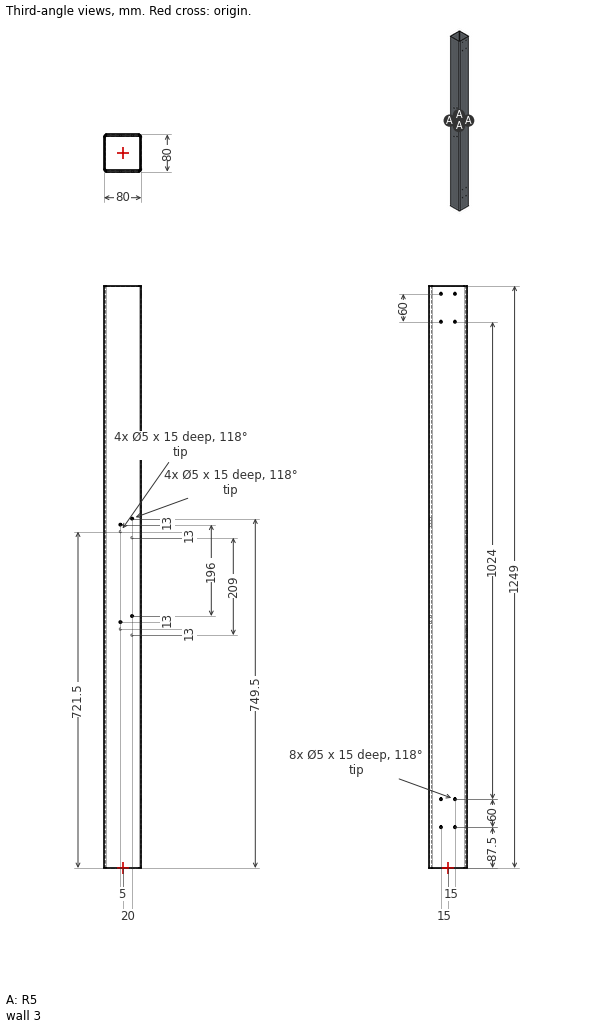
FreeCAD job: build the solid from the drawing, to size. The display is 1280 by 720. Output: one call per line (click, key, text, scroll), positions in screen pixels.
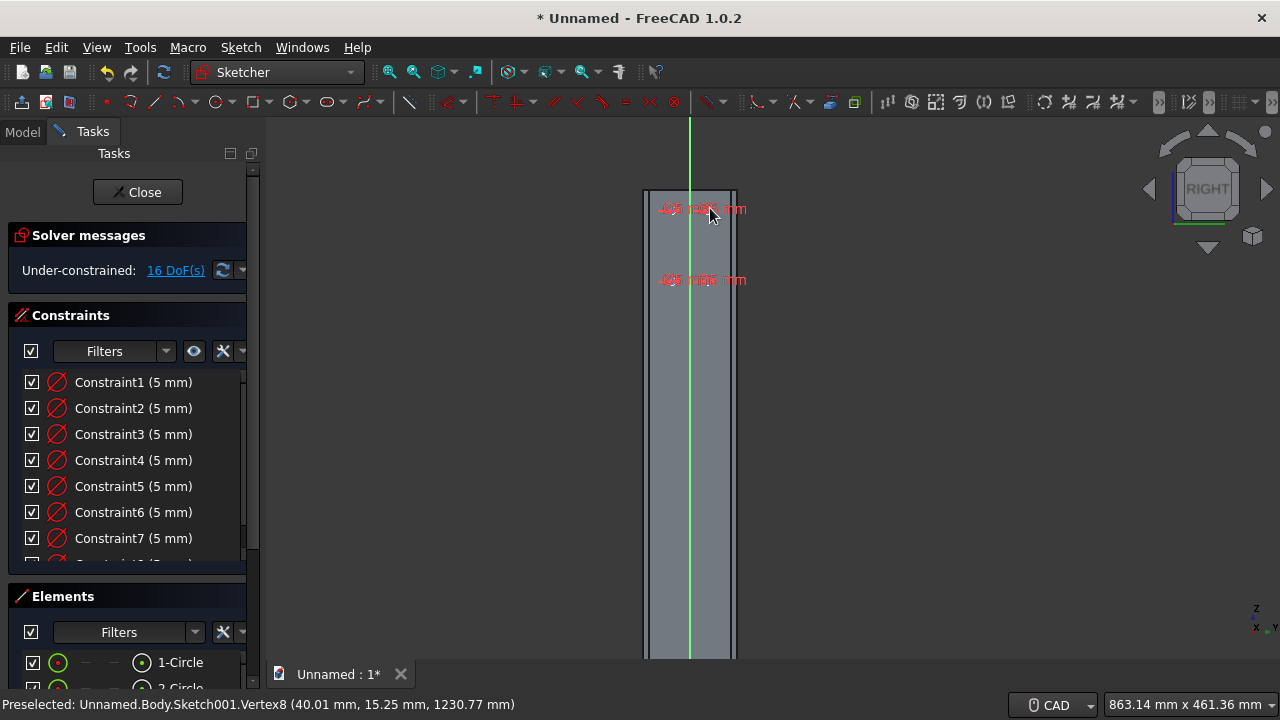
scroll(709, 210, down, 7)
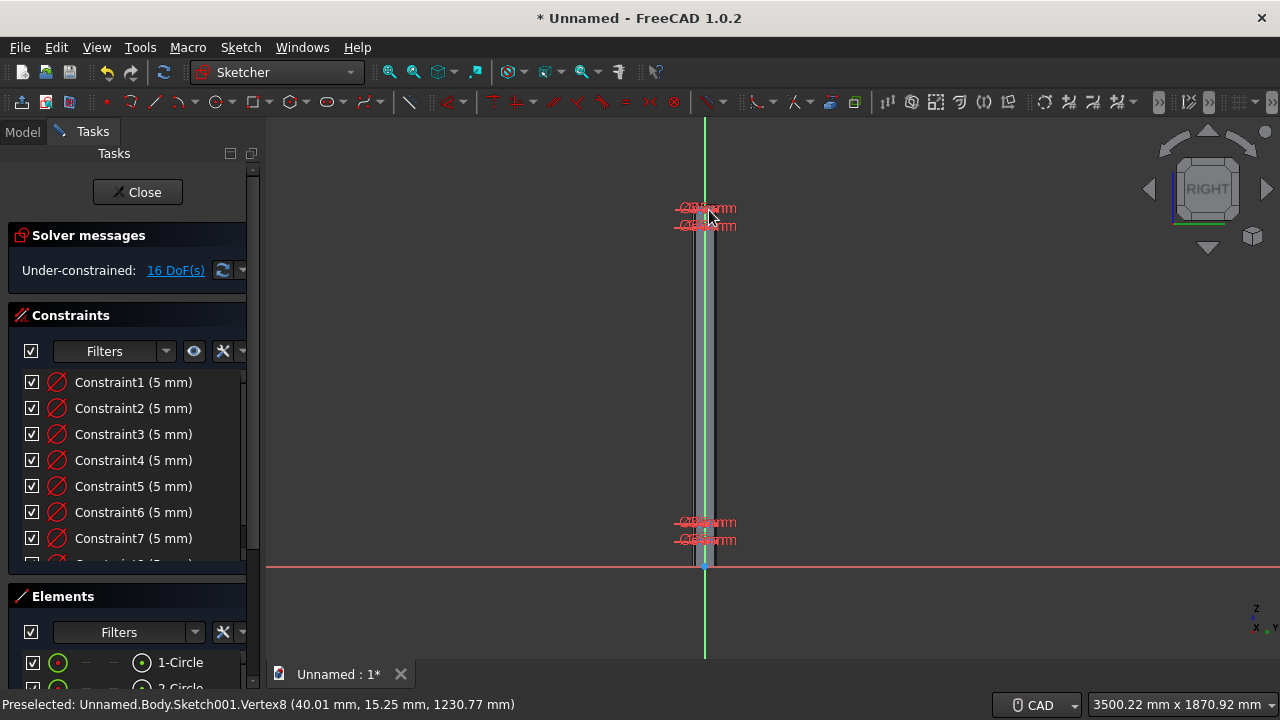
scroll(709, 525, up, 2)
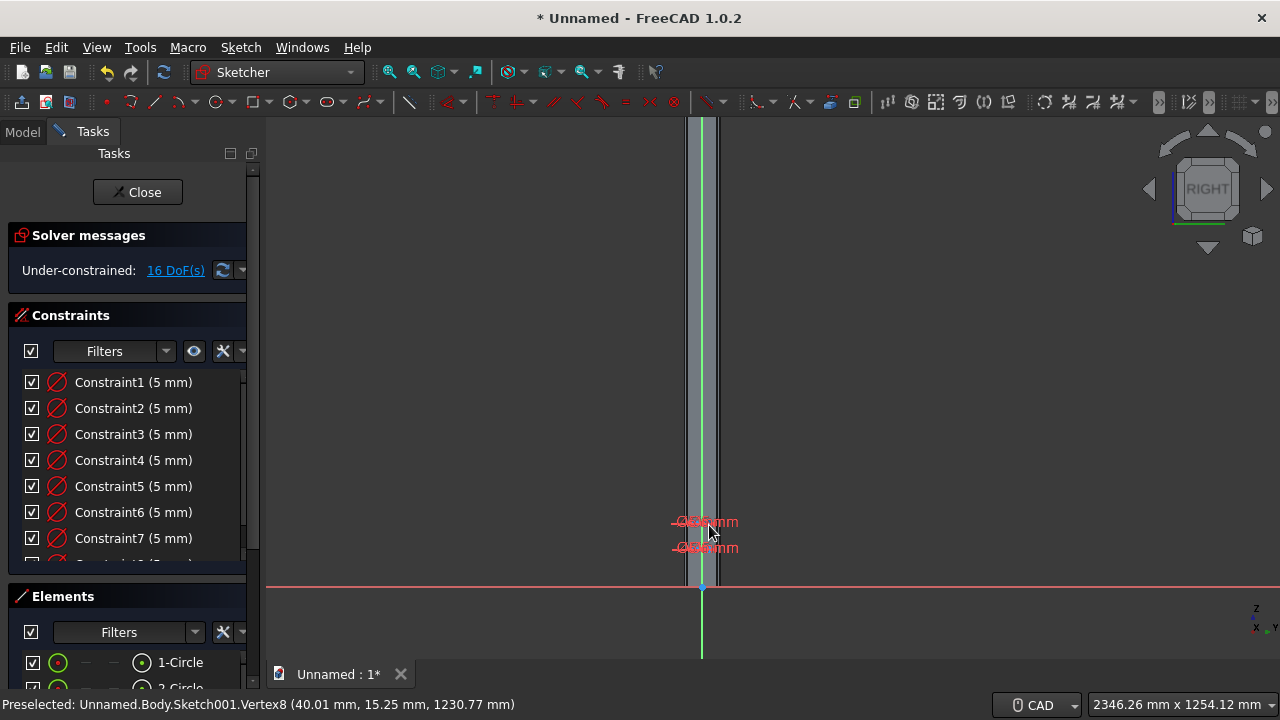
click(709, 524)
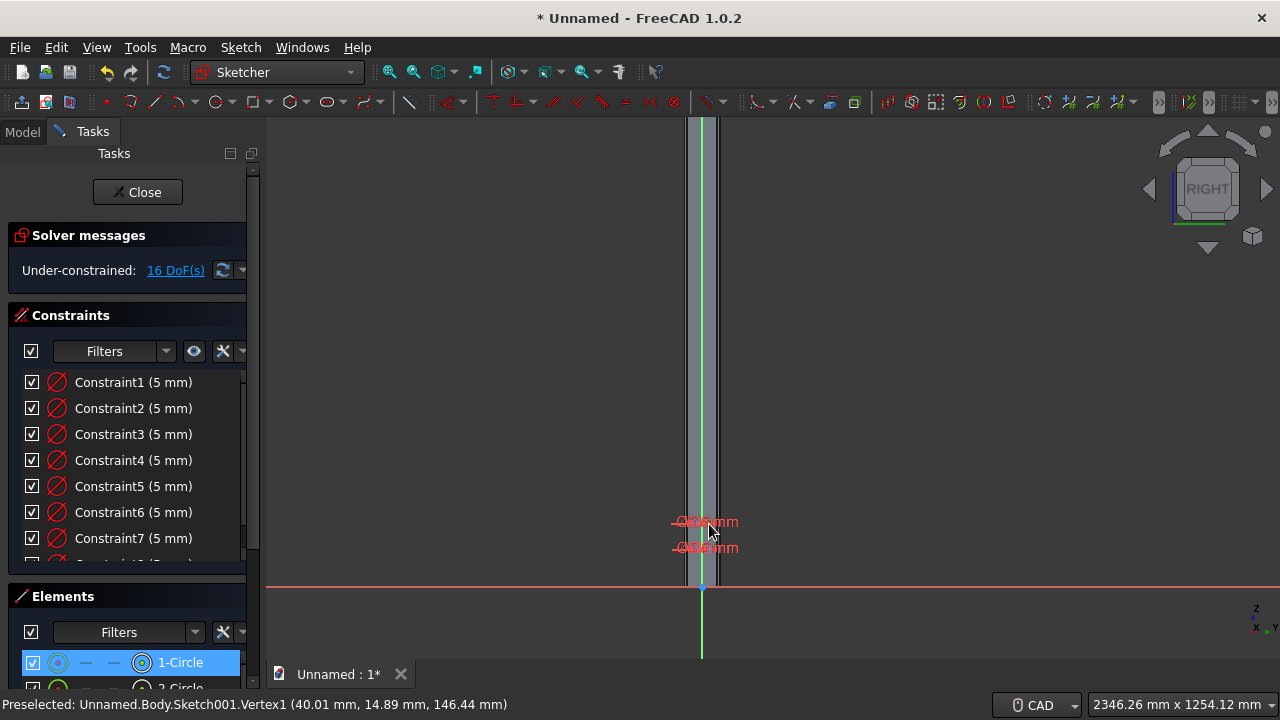
click(709, 550)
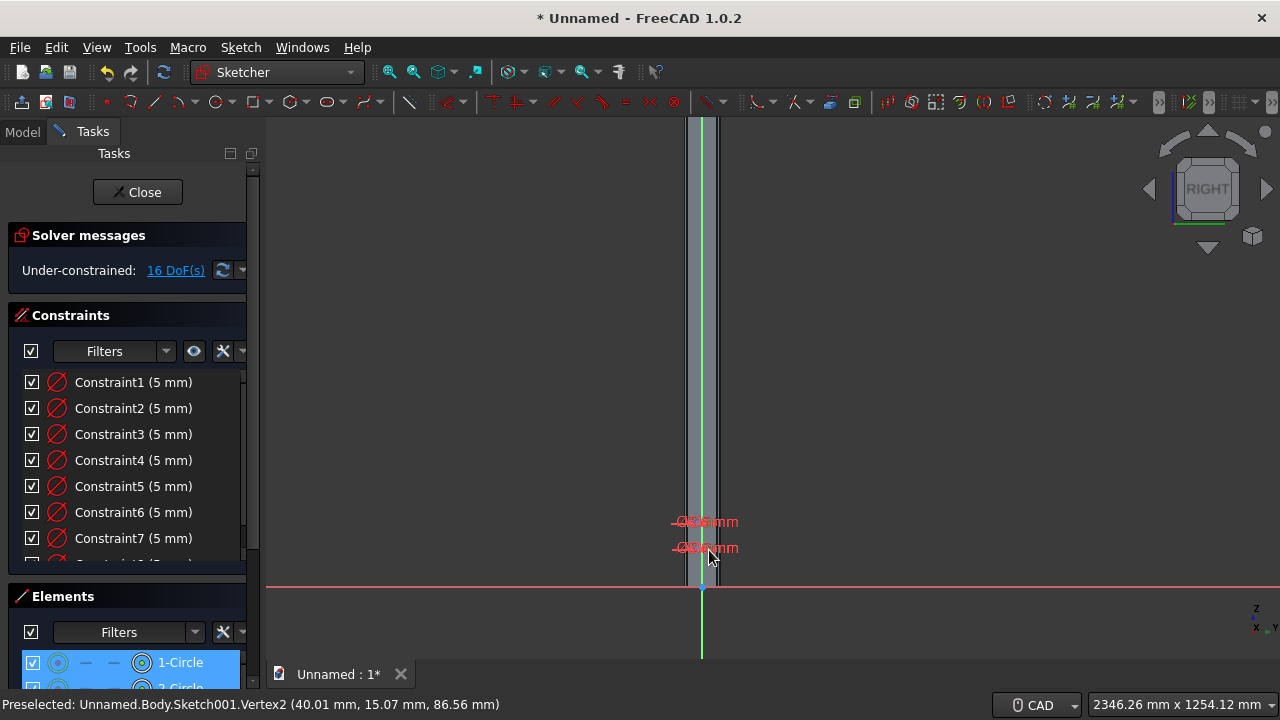
key(v)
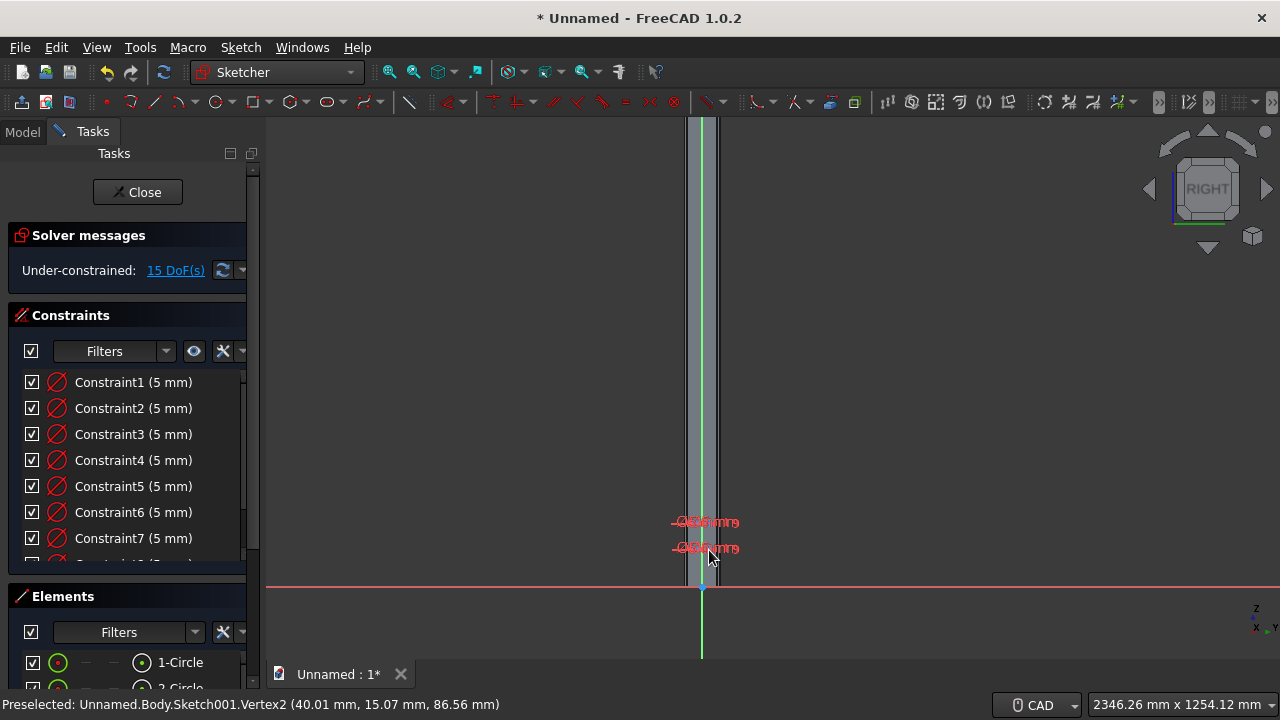
click(709, 550)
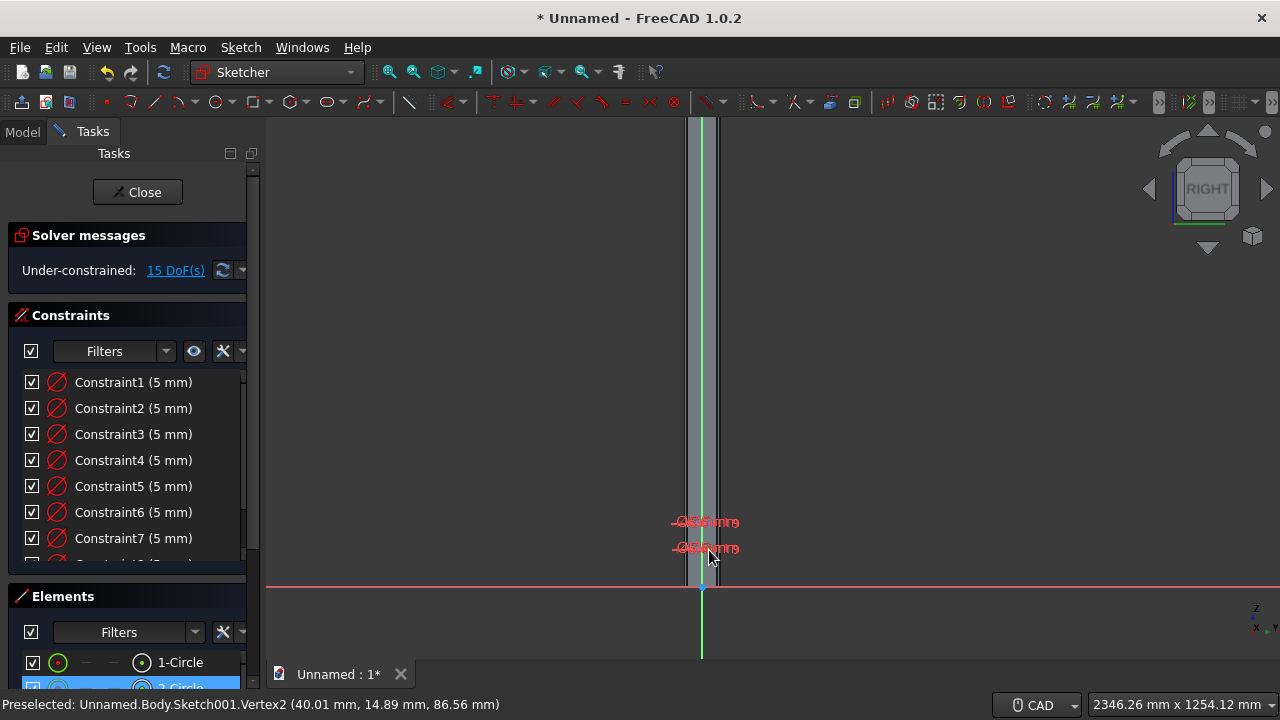
click(696, 550)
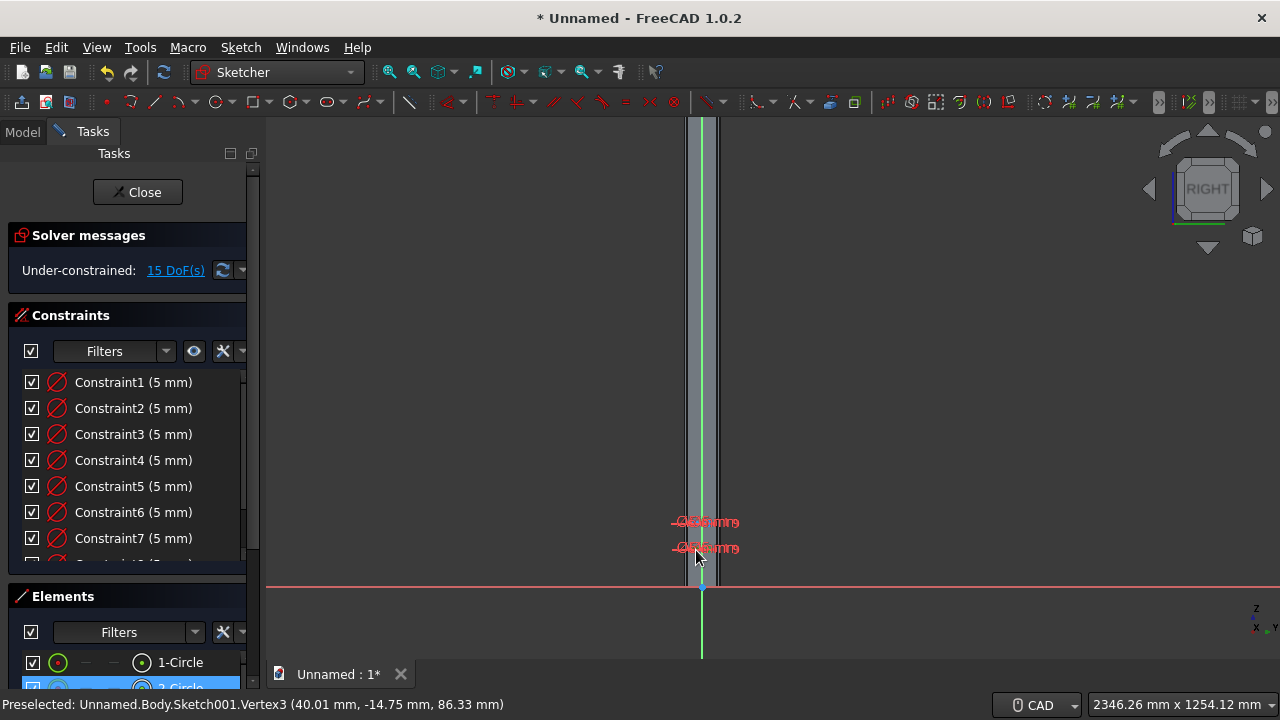
click(536, 102)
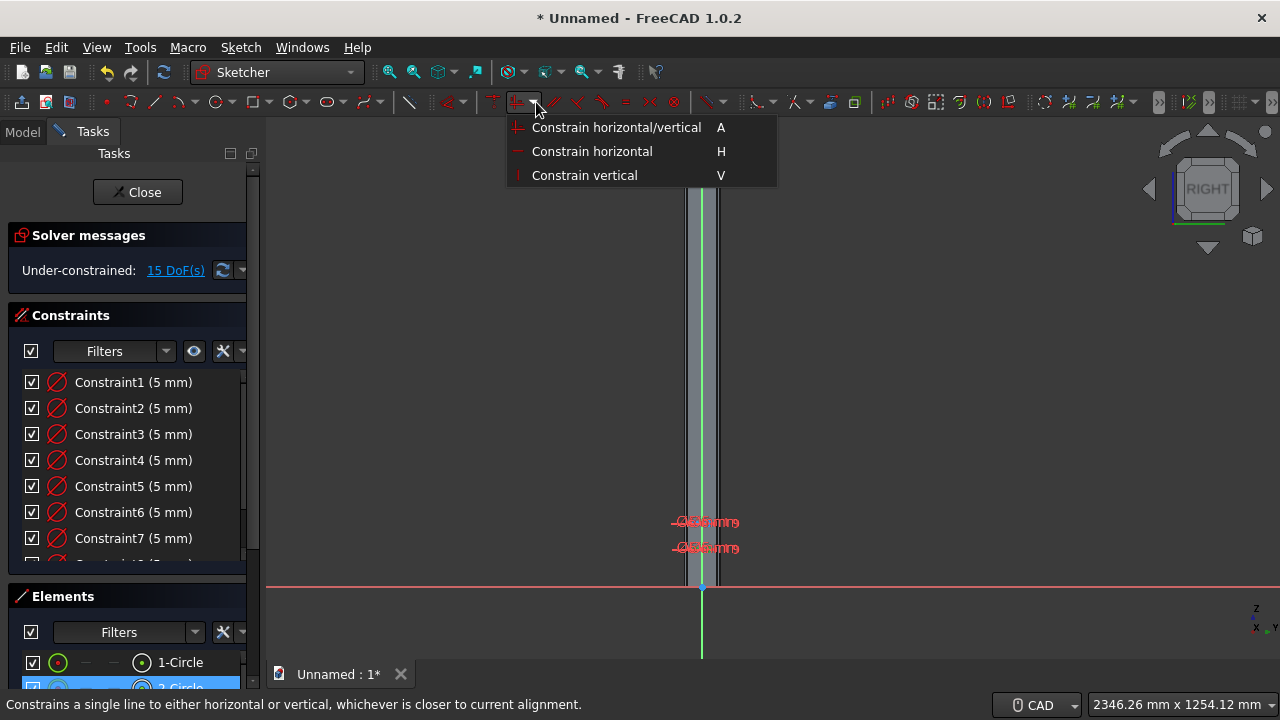
click(642, 151)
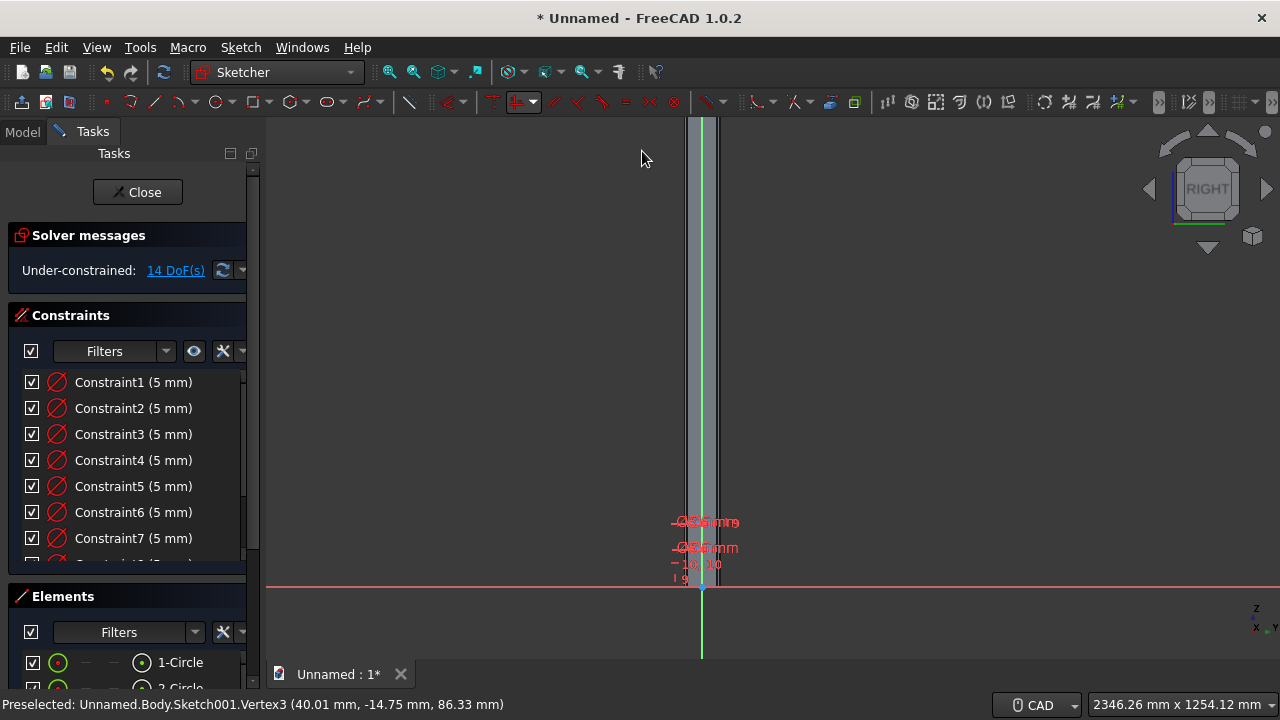
click(696, 550)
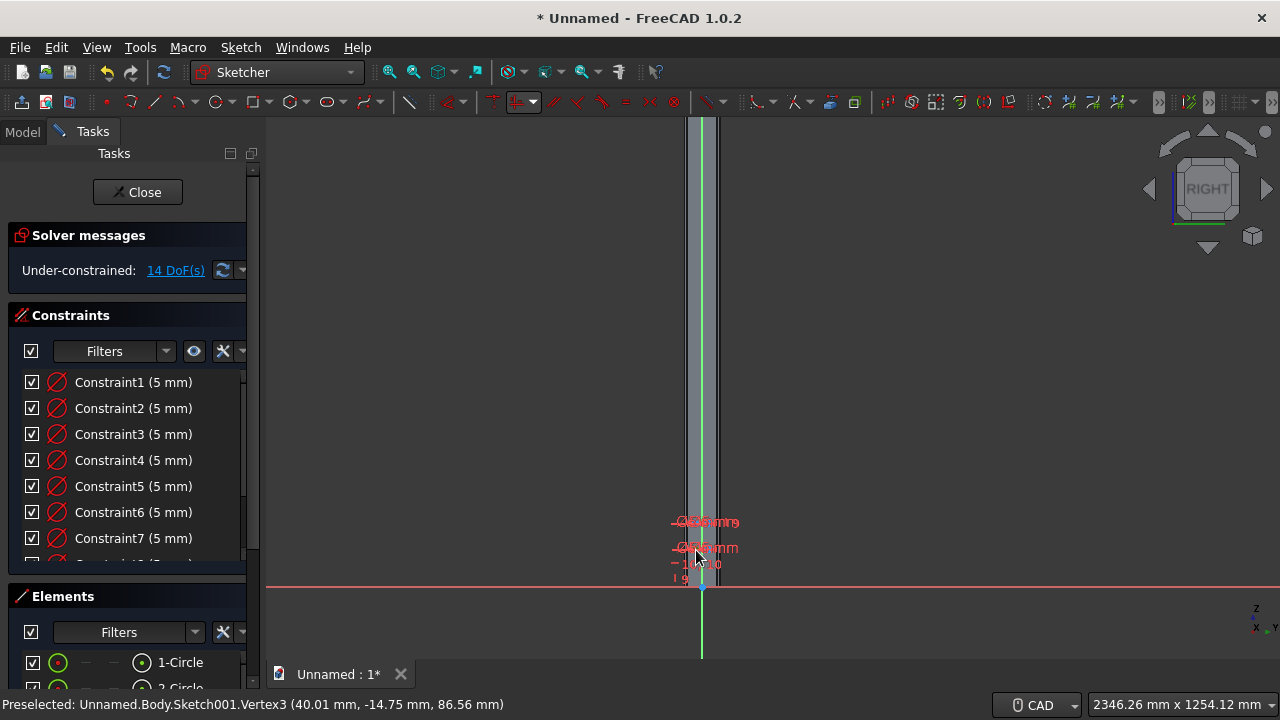
click(696, 524)